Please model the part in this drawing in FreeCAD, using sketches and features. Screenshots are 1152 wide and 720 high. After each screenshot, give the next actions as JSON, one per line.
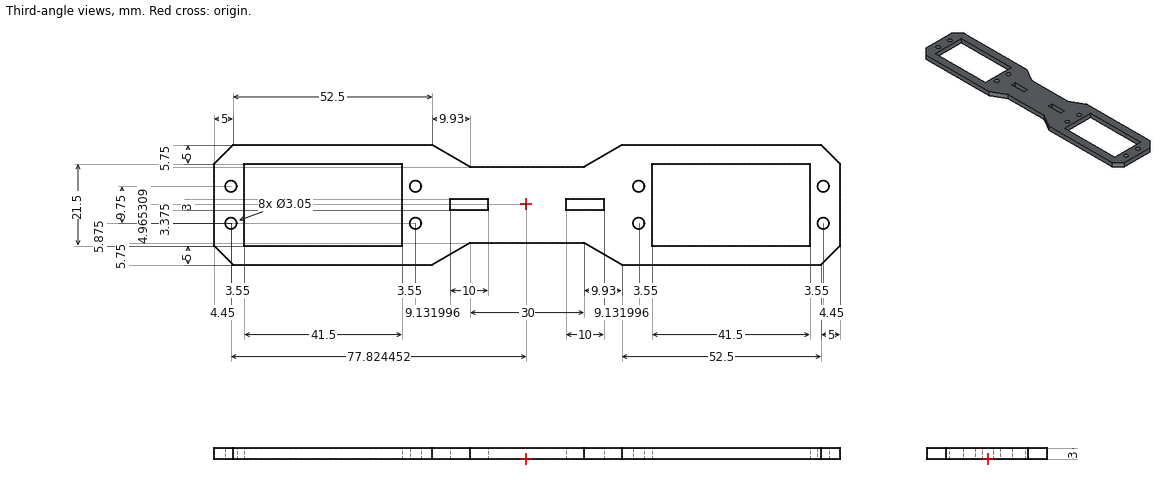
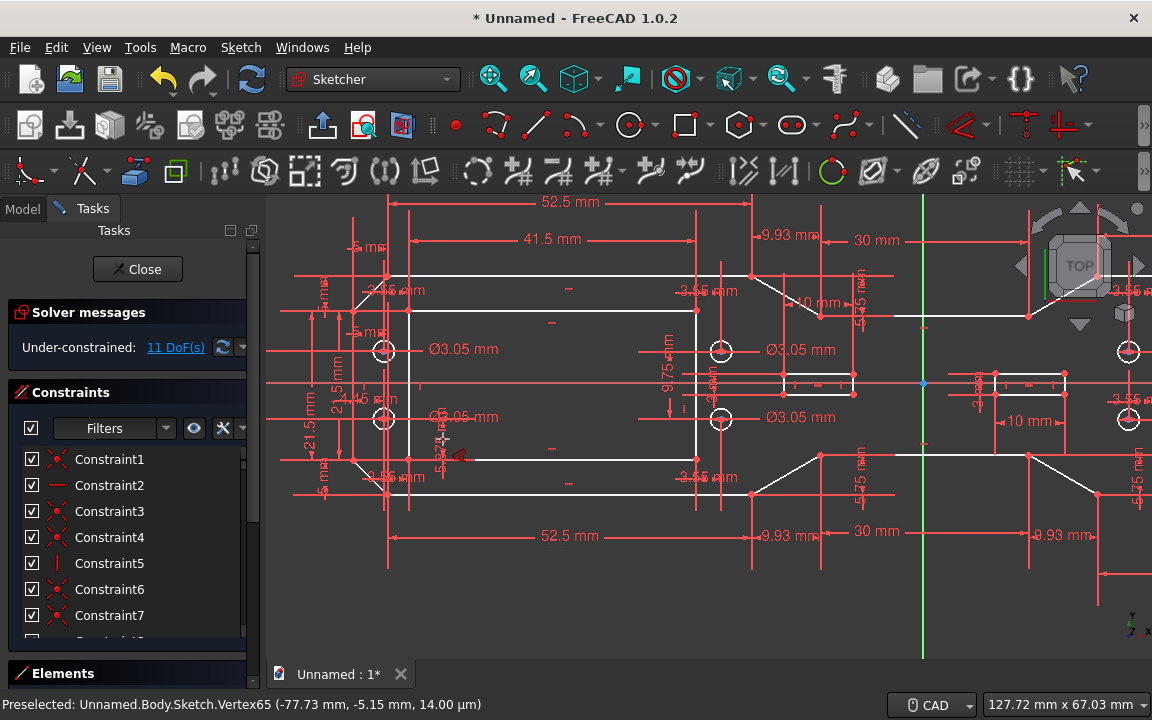
{"action": "left_click", "coordinate": [353, 460]}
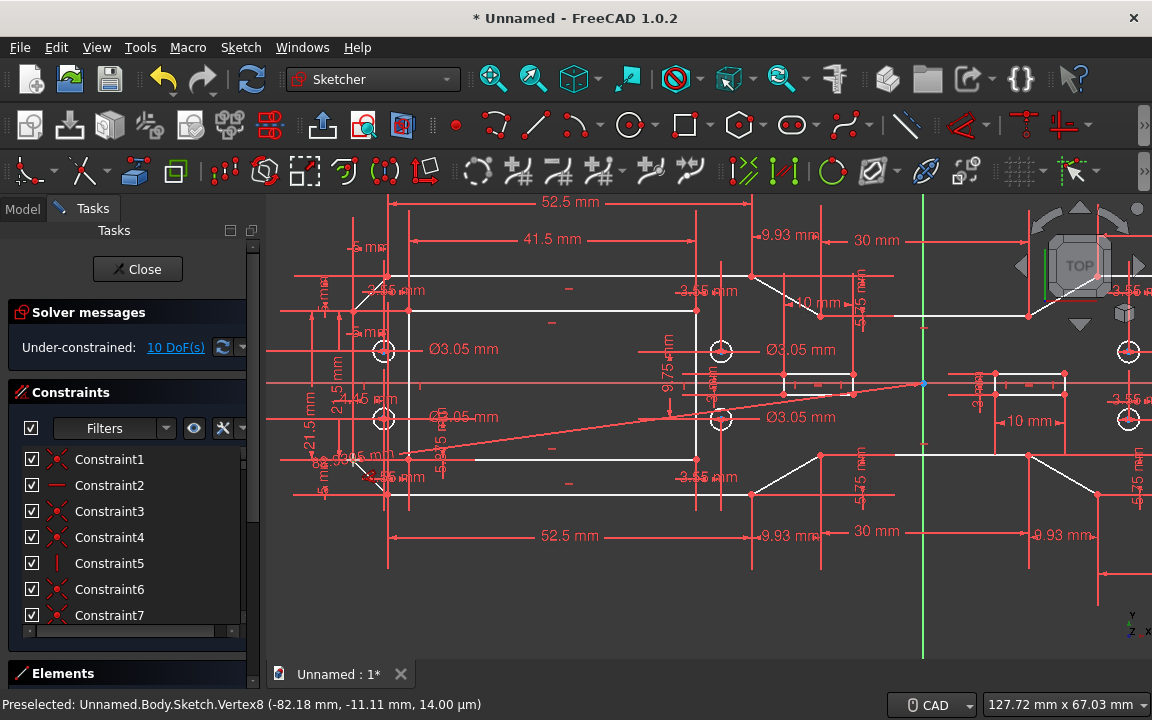
{"action": "left_click", "coordinate": [384, 419]}
{"action": "left_click", "coordinate": [319, 449]}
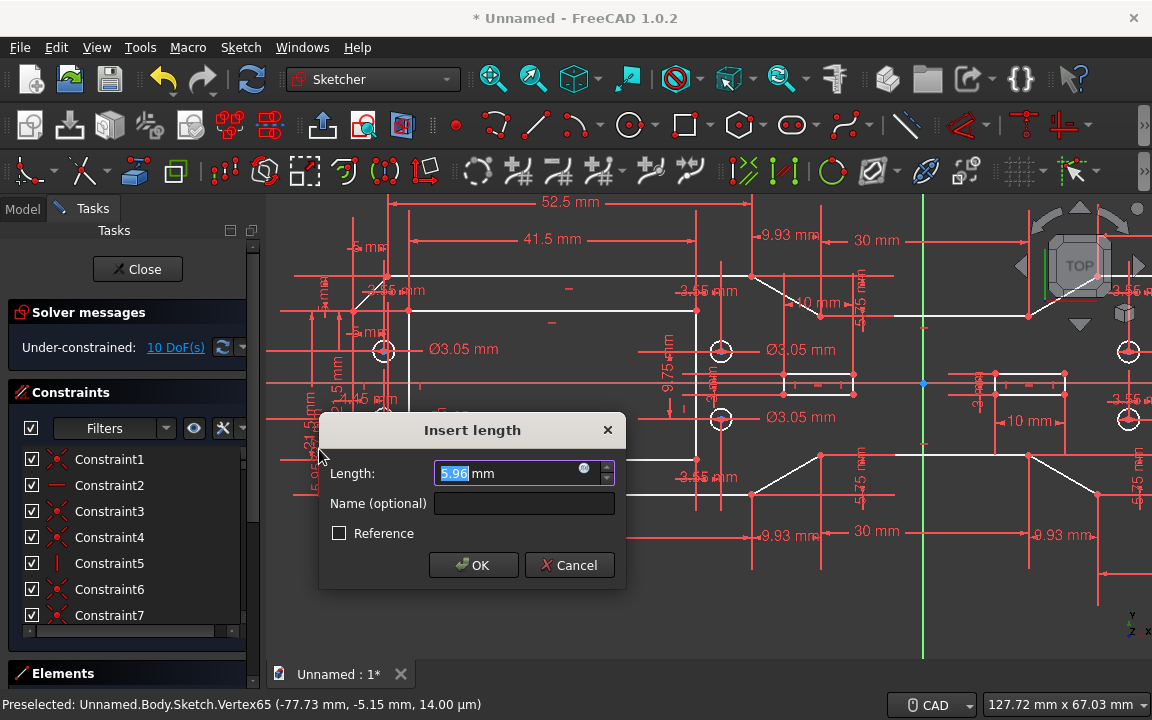
{"action": "type", "text": "5.875"}
{"action": "key", "text": "Return"}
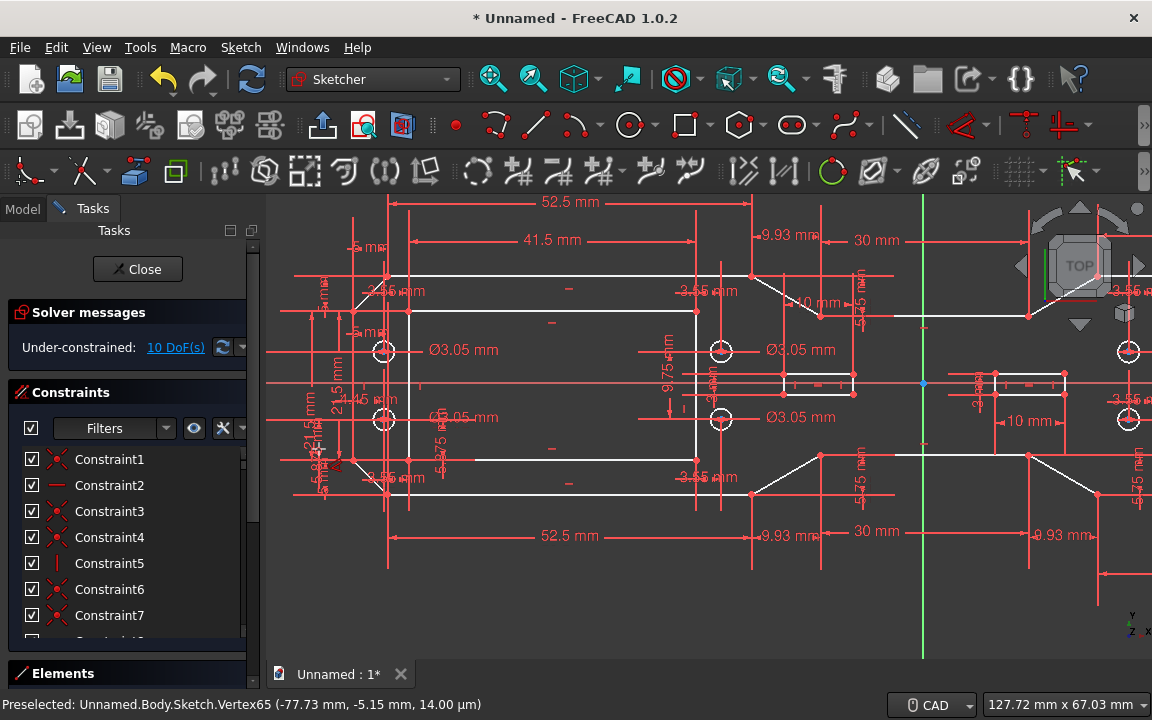
{"action": "left_click", "coordinate": [696, 460]}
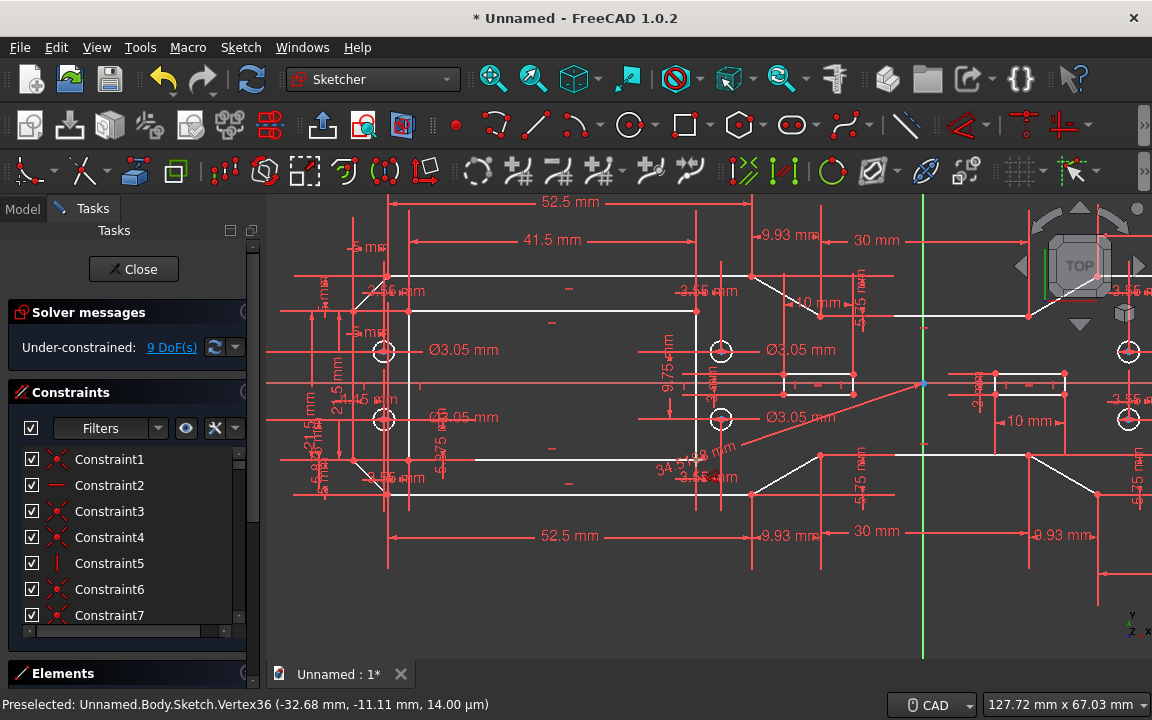
{"action": "left_click", "coordinate": [721, 419]}
{"action": "left_click", "coordinate": [662, 440]}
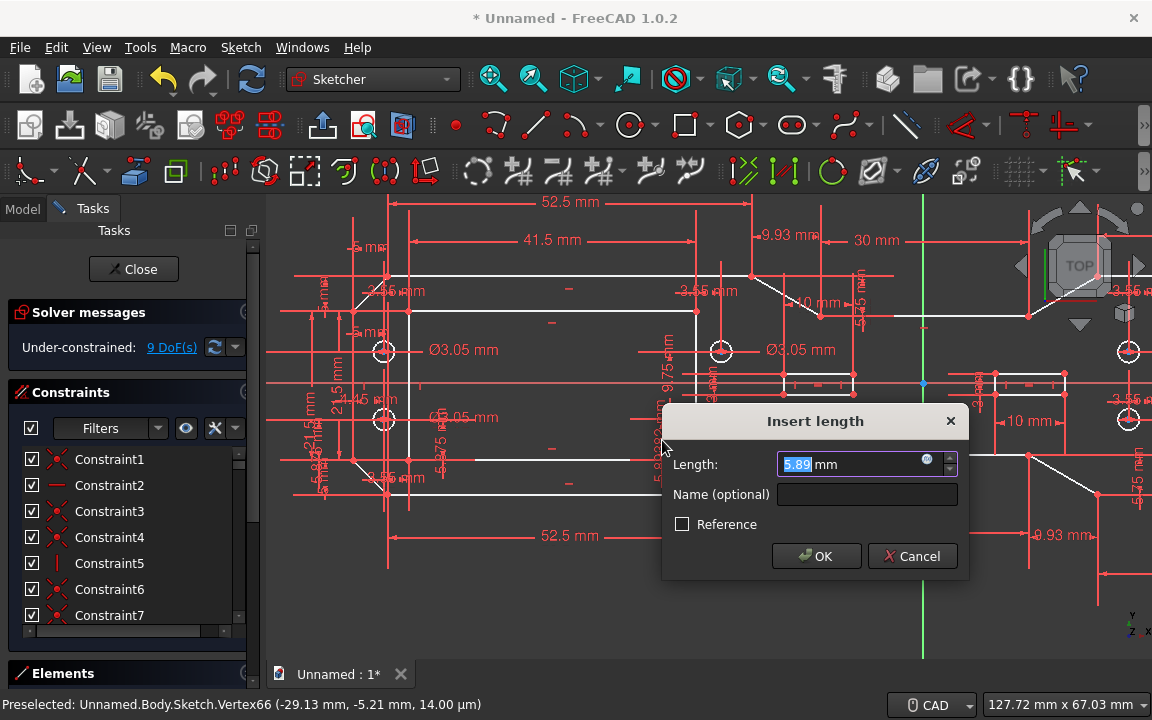
{"action": "type", "text": "5.875"}
{"action": "key", "text": "Return"}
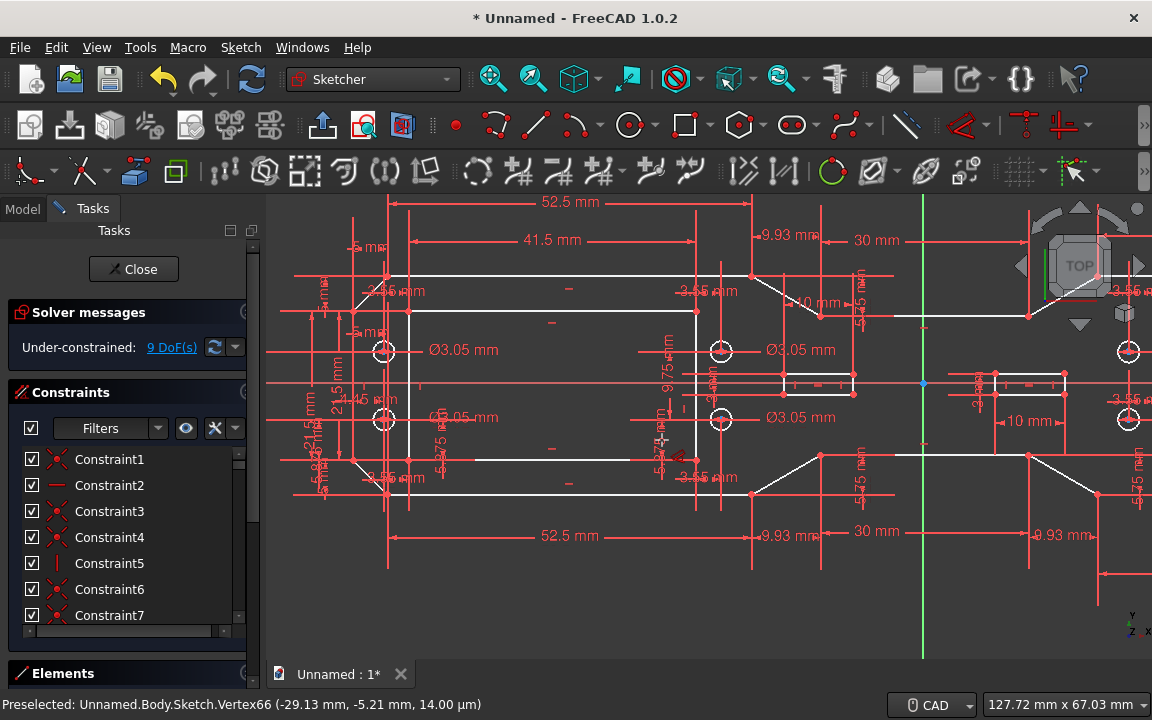
{"action": "scroll", "coordinate": [784, 395], "scroll_direction": "up", "scroll_amount": 3}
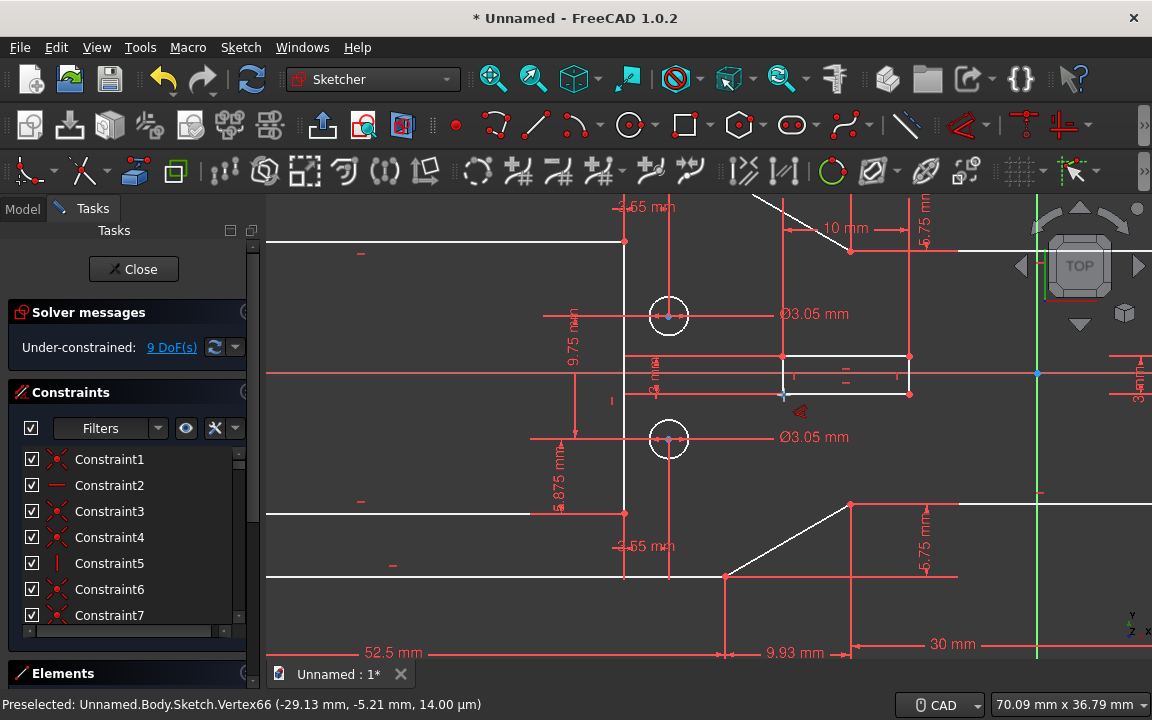
{"action": "left_click", "coordinate": [783, 394]}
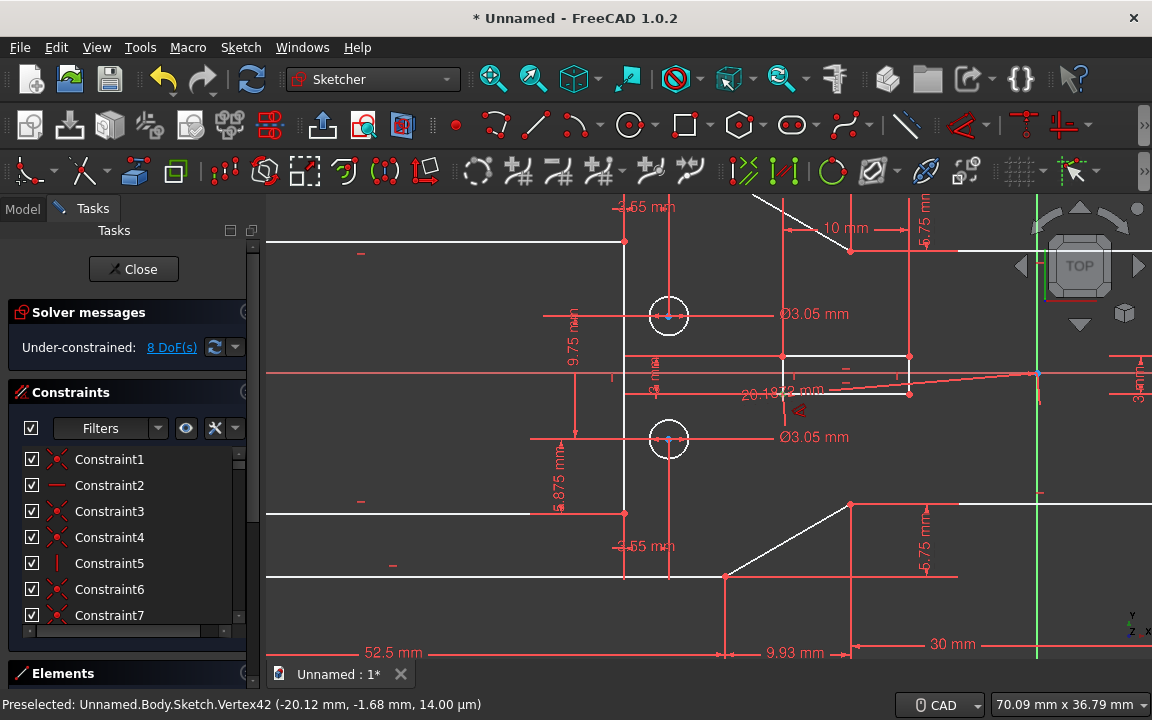
{"action": "left_click", "coordinate": [669, 439]}
{"action": "left_click", "coordinate": [817, 417]}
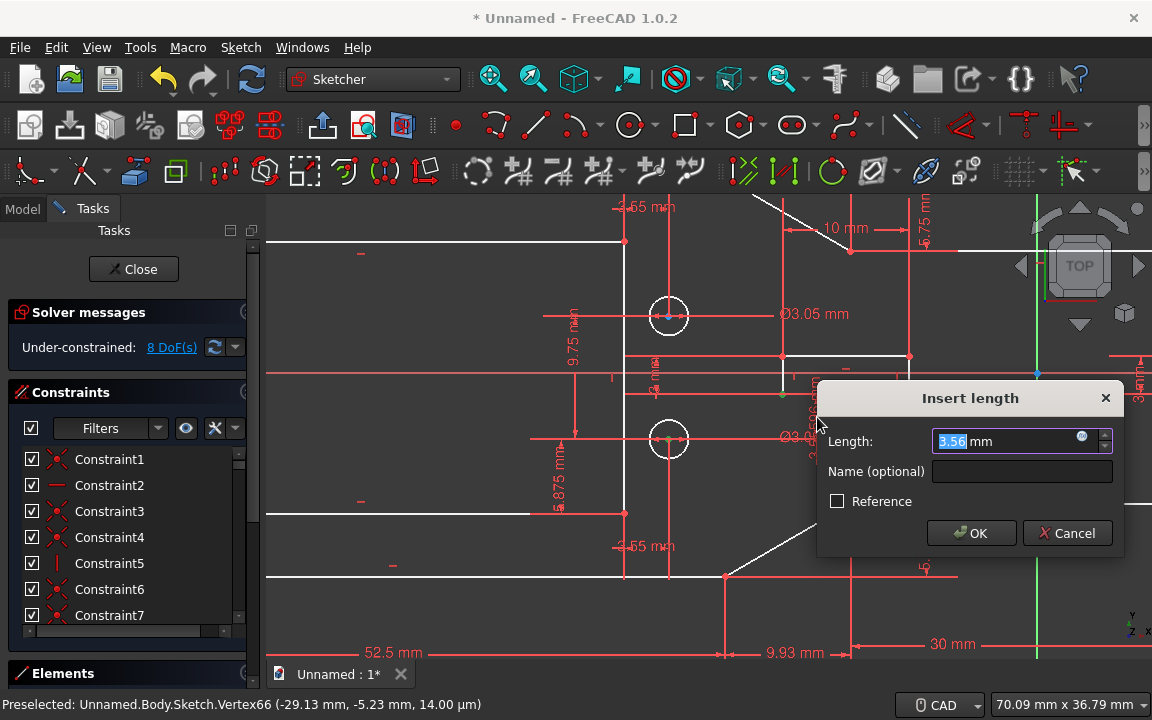
{"action": "type", "text": "3.375"}
{"action": "key", "text": "Return"}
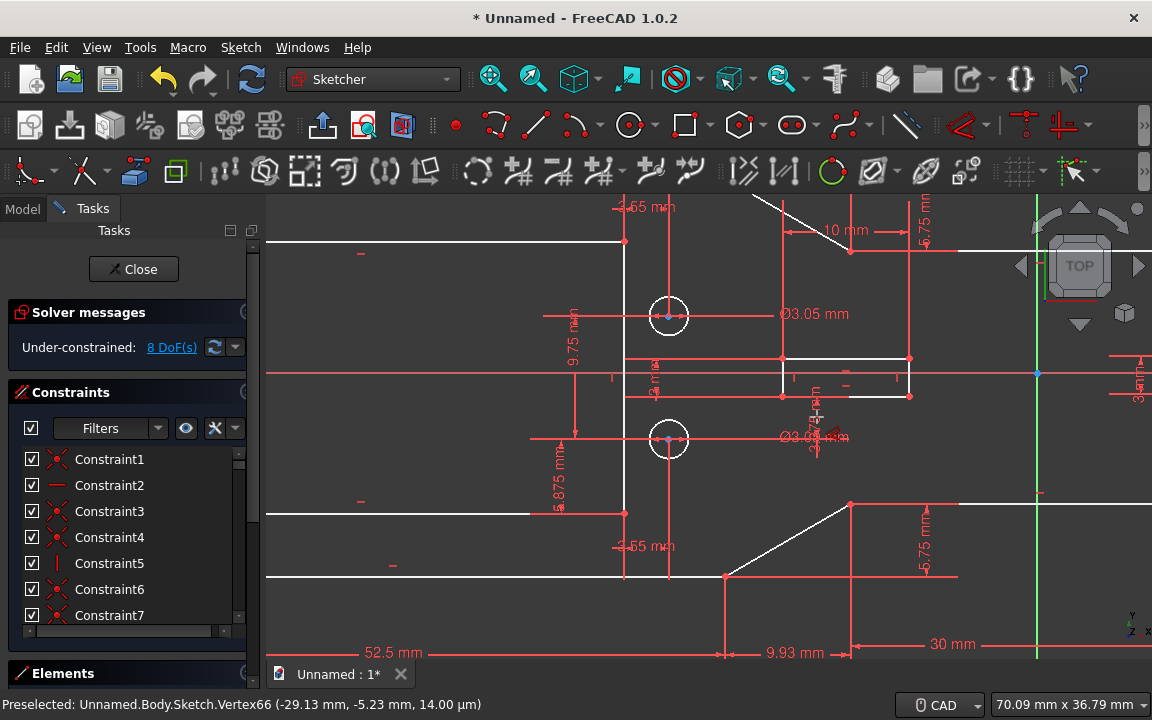
{"action": "scroll", "coordinate": [510, 444], "scroll_direction": "down", "scroll_amount": 7}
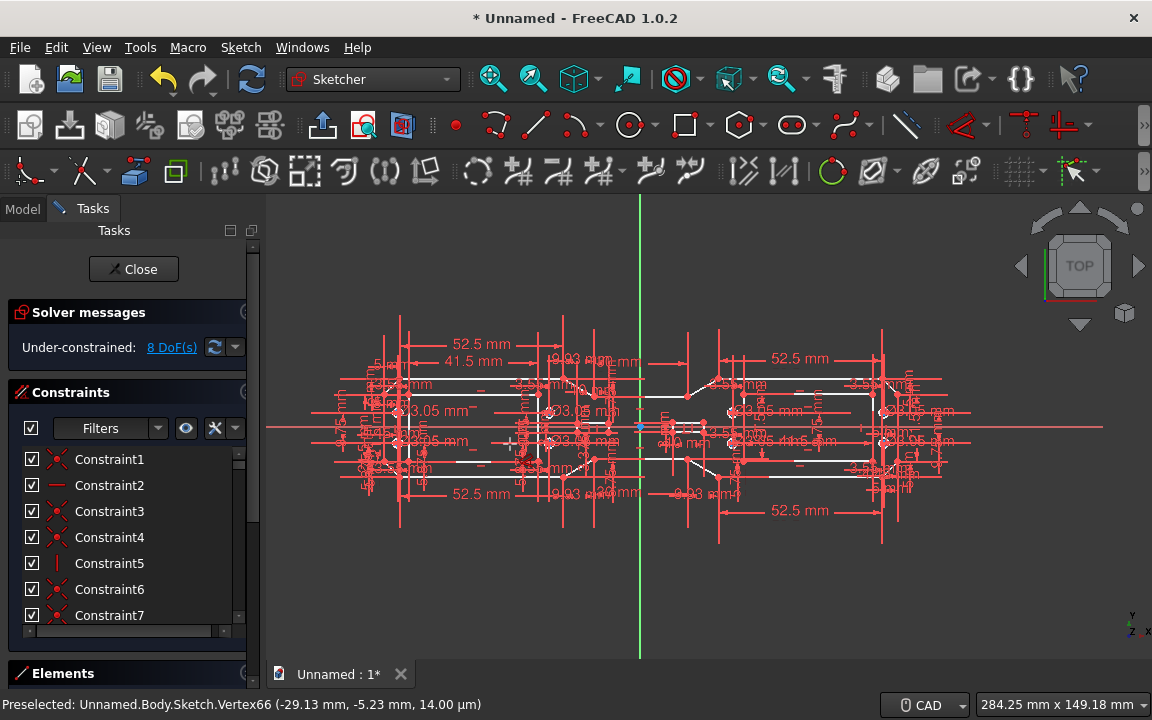
{"action": "scroll", "coordinate": [744, 461], "scroll_direction": "up", "scroll_amount": 4}